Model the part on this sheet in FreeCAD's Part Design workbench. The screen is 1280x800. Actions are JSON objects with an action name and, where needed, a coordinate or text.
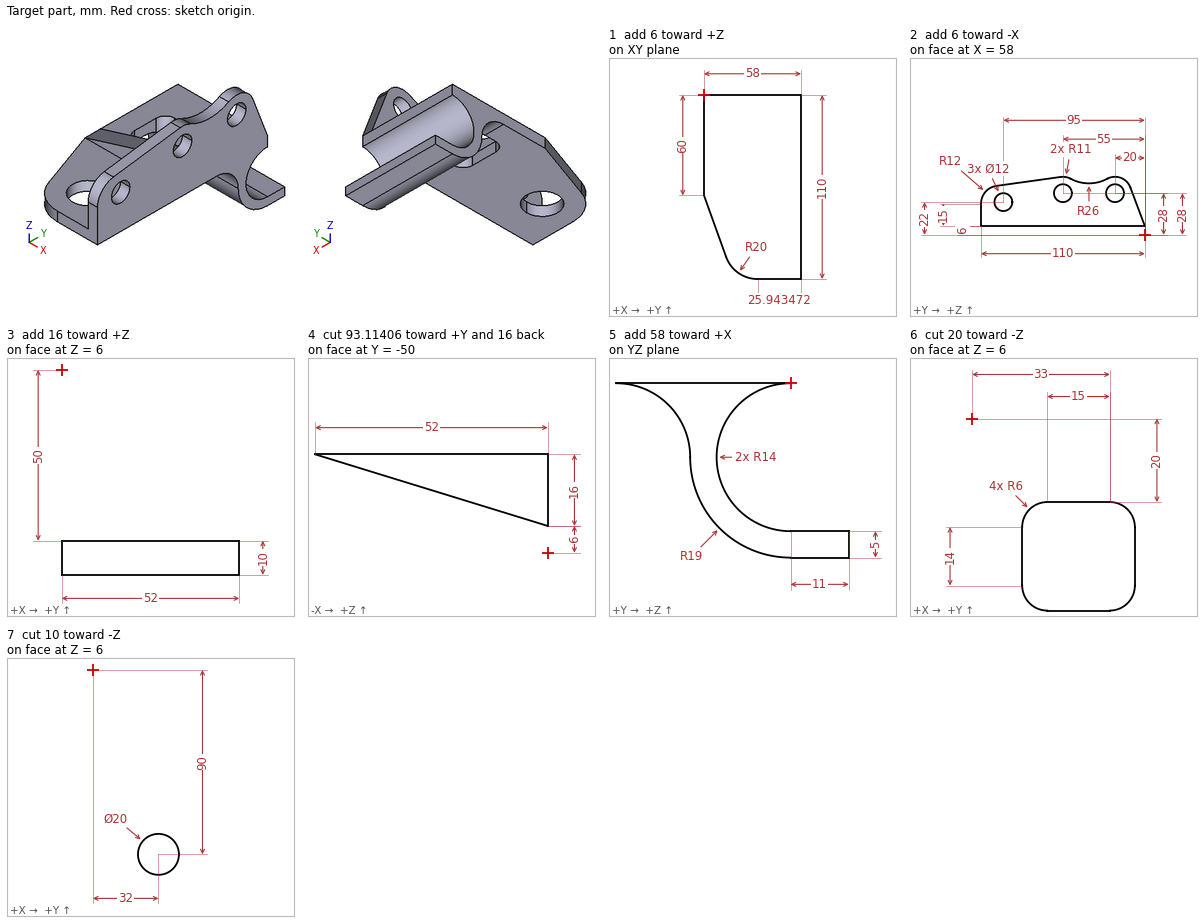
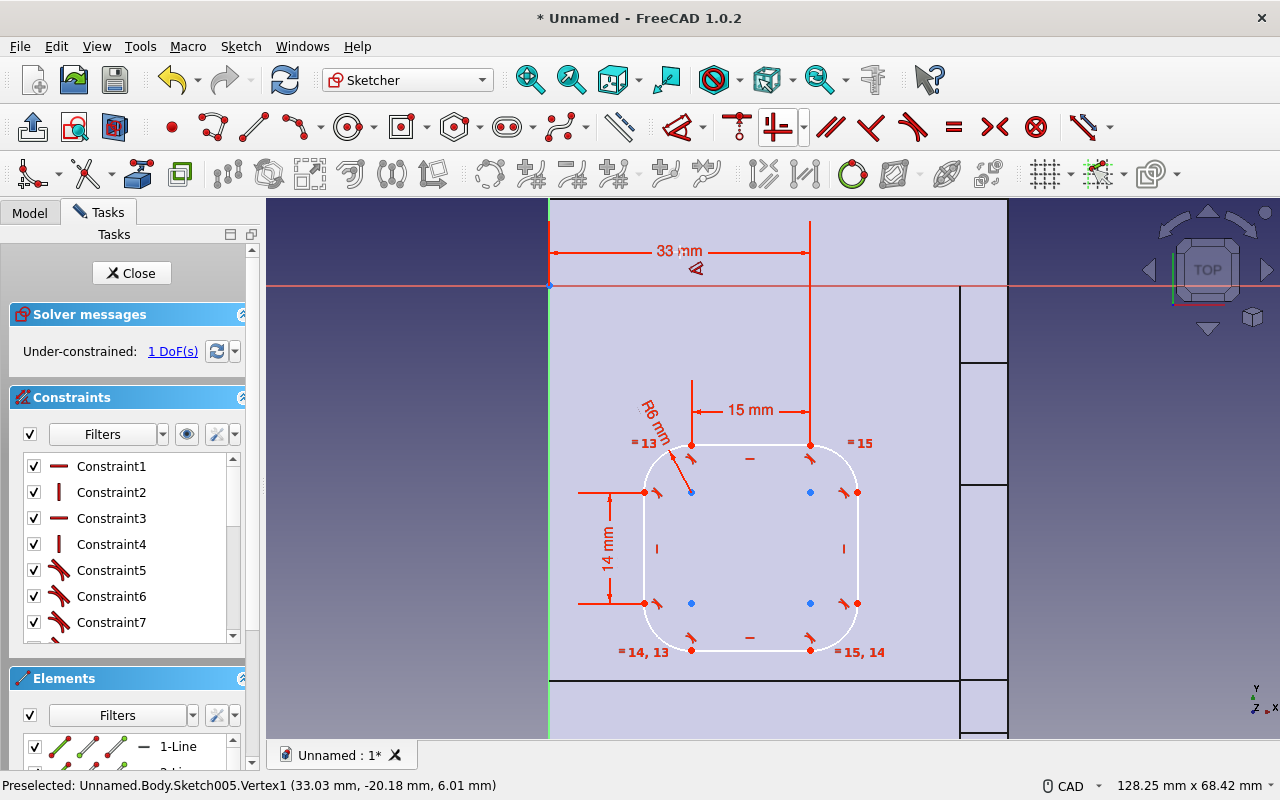
{"action": "left_click", "coordinate": [810, 445]}
{"action": "left_click", "coordinate": [515, 366]}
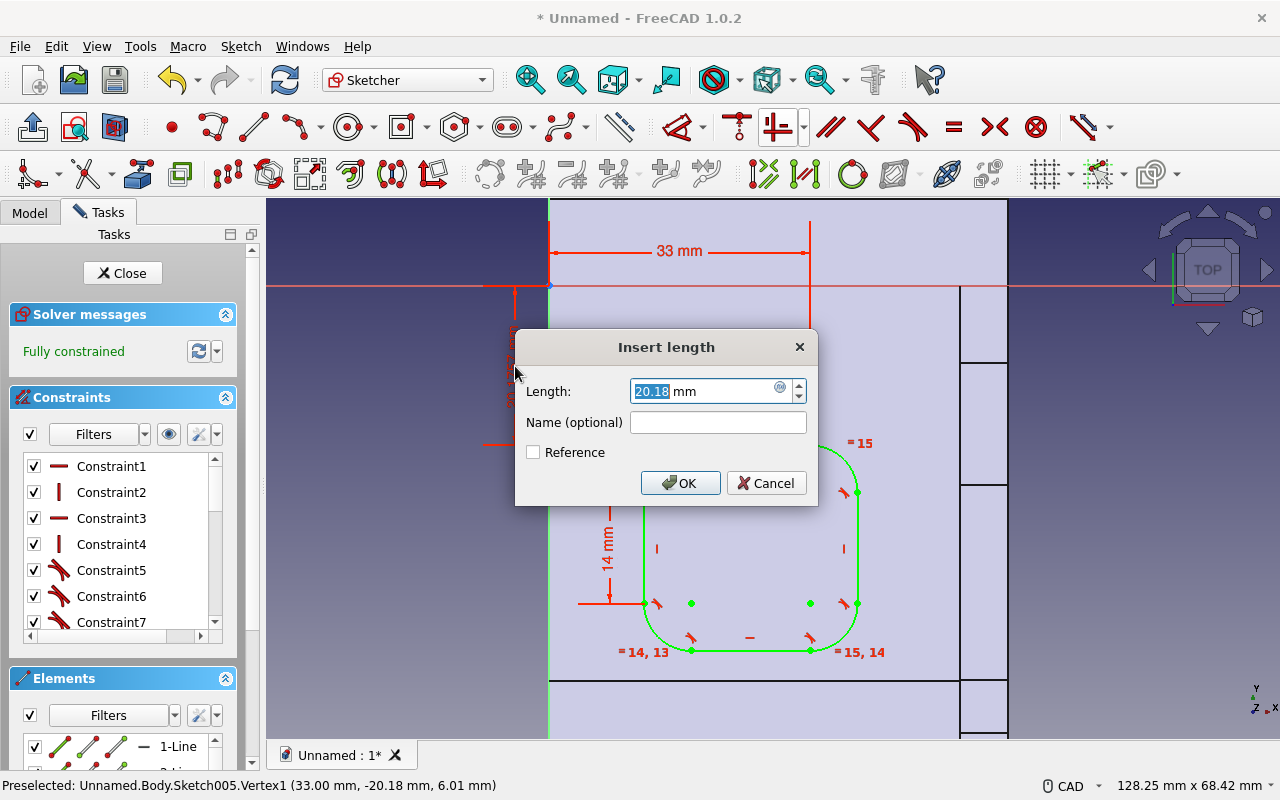
{"action": "type", "text": "20"}
{"action": "key", "text": "Return"}
{"action": "key", "text": "Escape"}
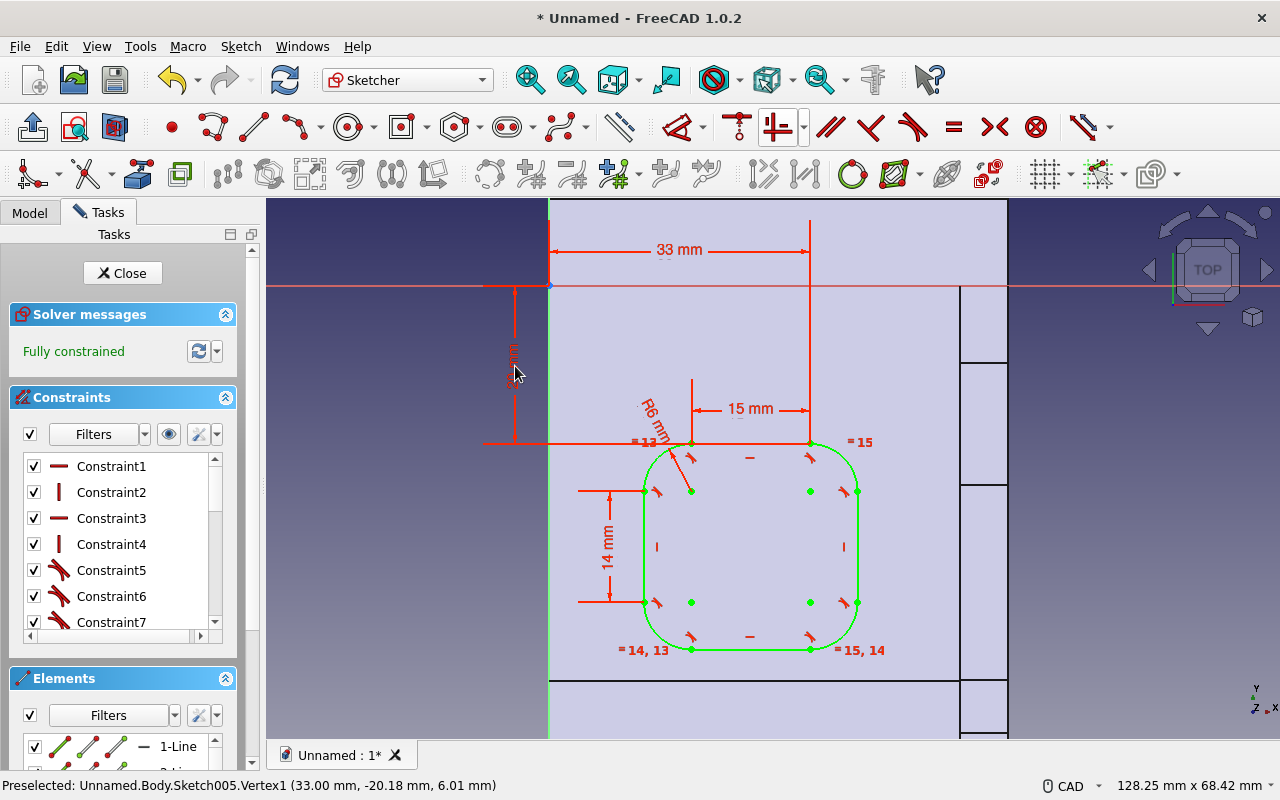
{"action": "left_click", "coordinate": [123, 273]}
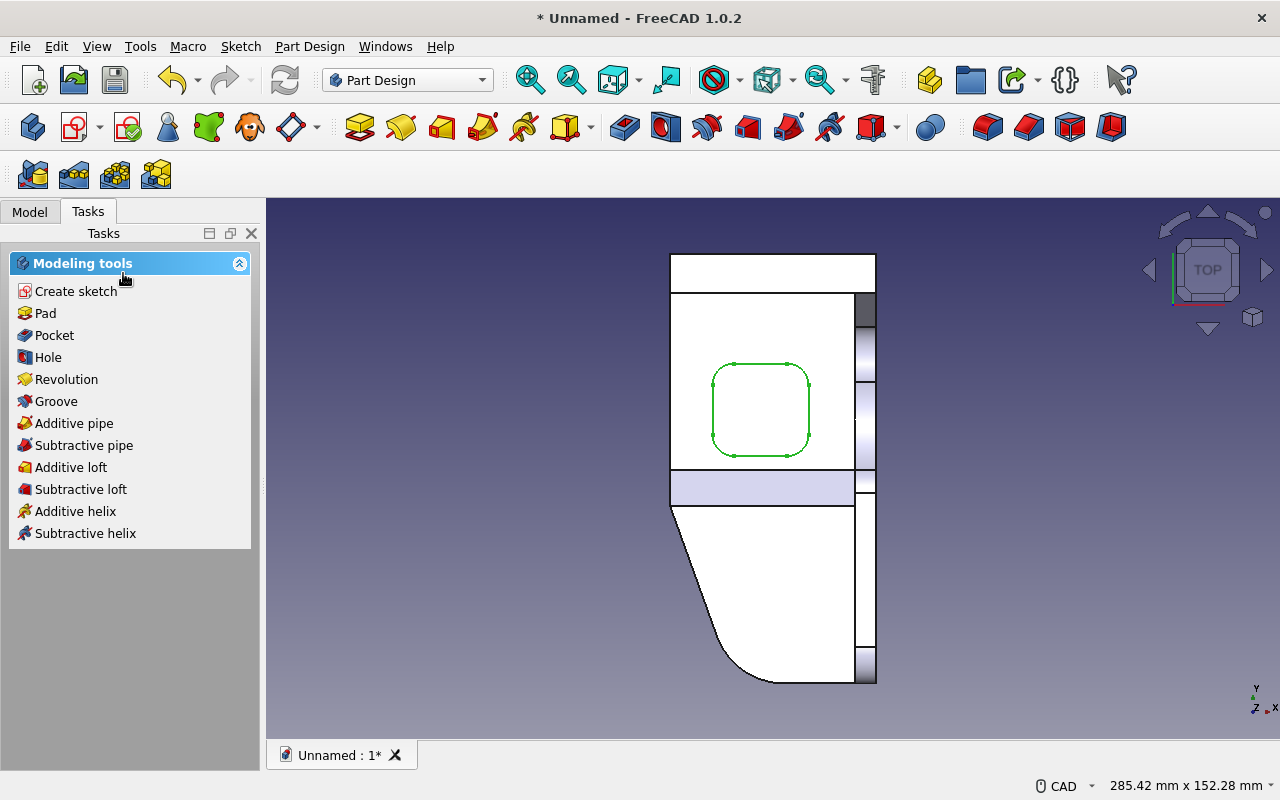
{"action": "left_click", "coordinate": [625, 128]}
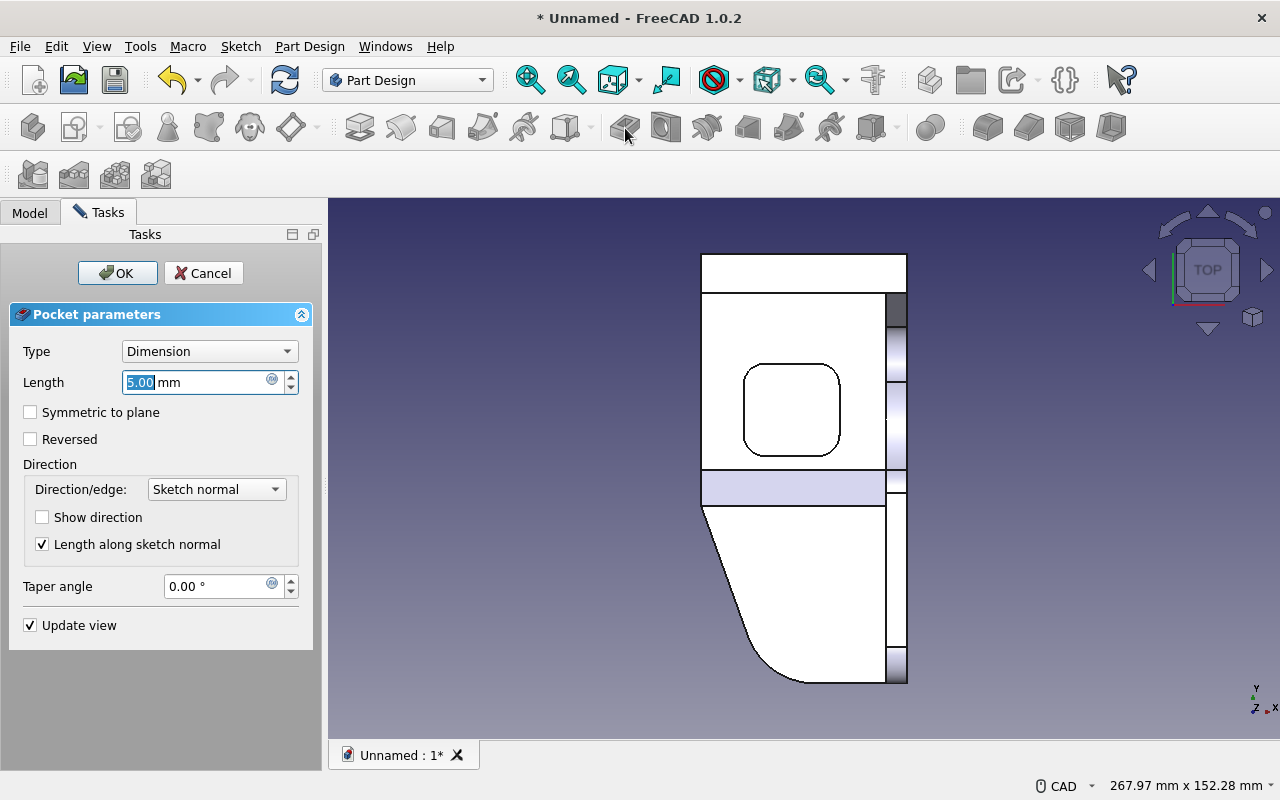
{"action": "type", "text": "20"}
{"action": "key", "text": "Tab"}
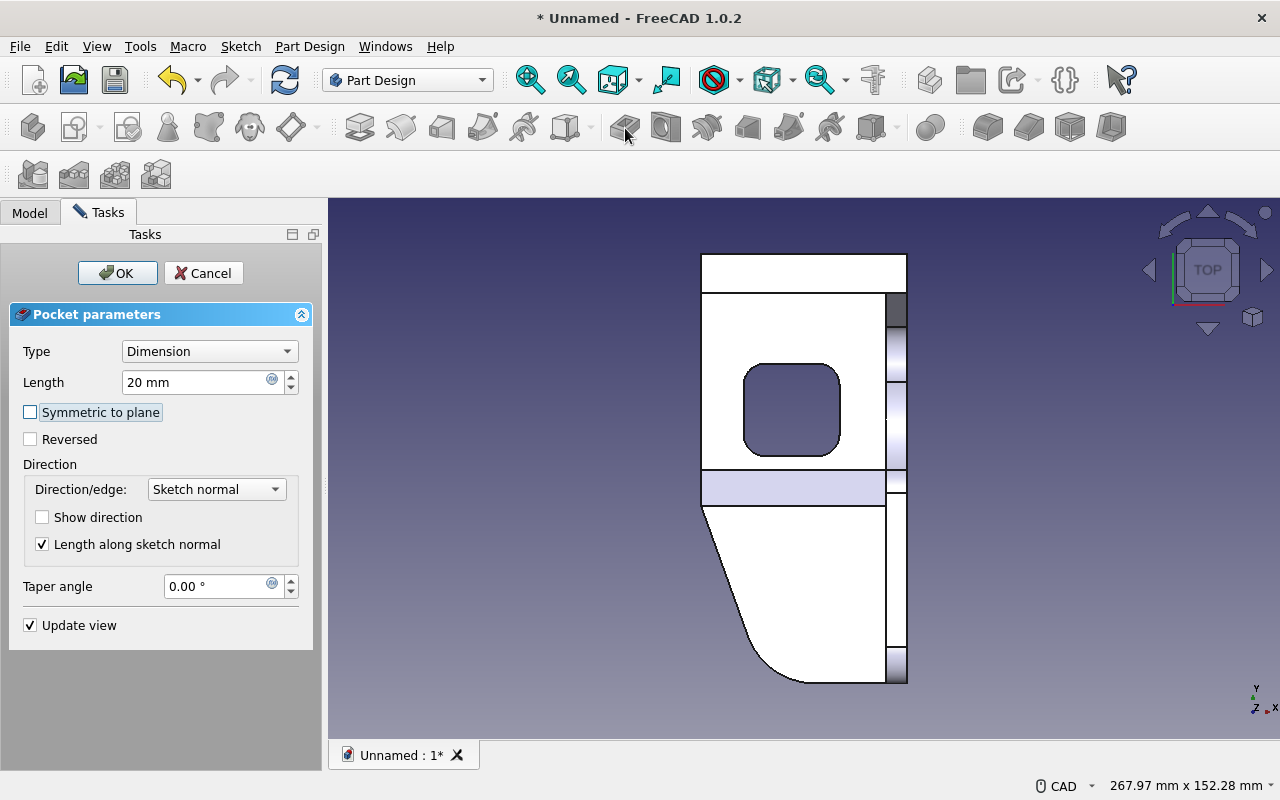
{"action": "left_click", "coordinate": [118, 273]}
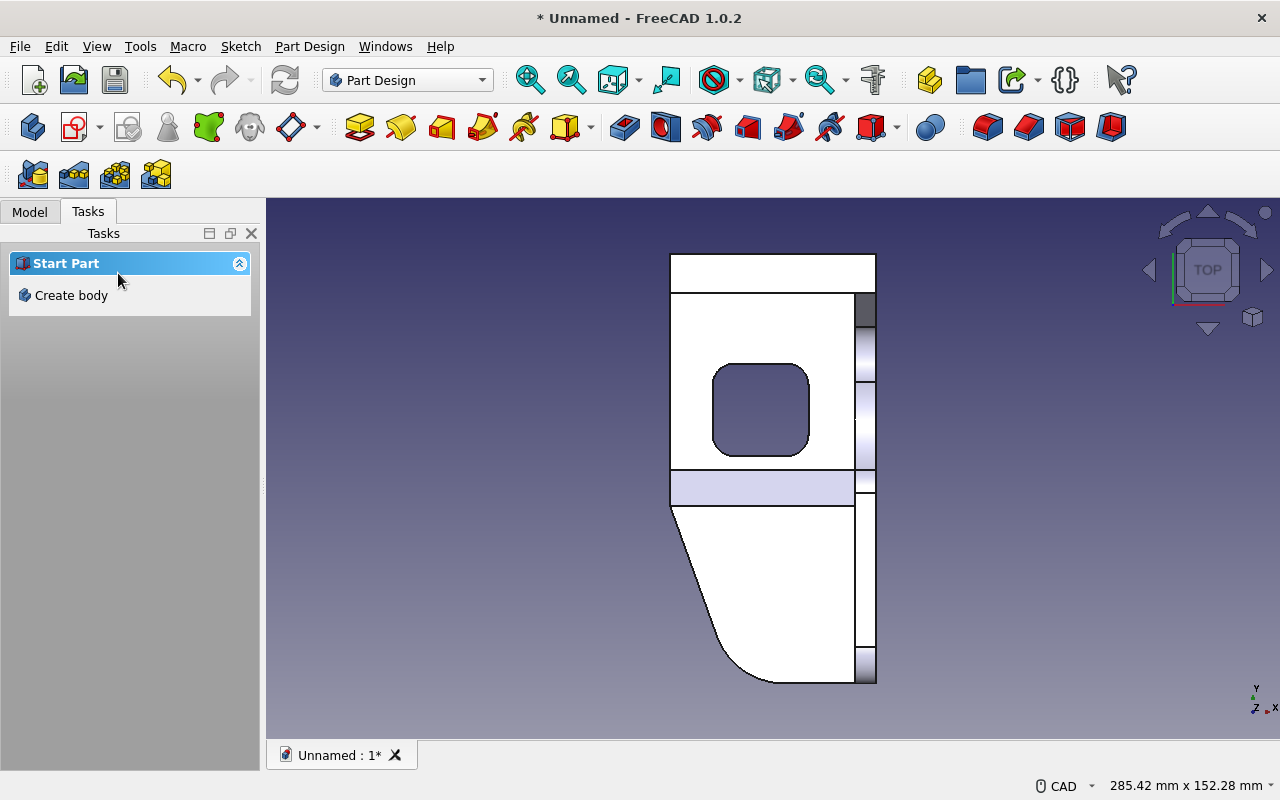
{"action": "left_click", "coordinate": [789, 594]}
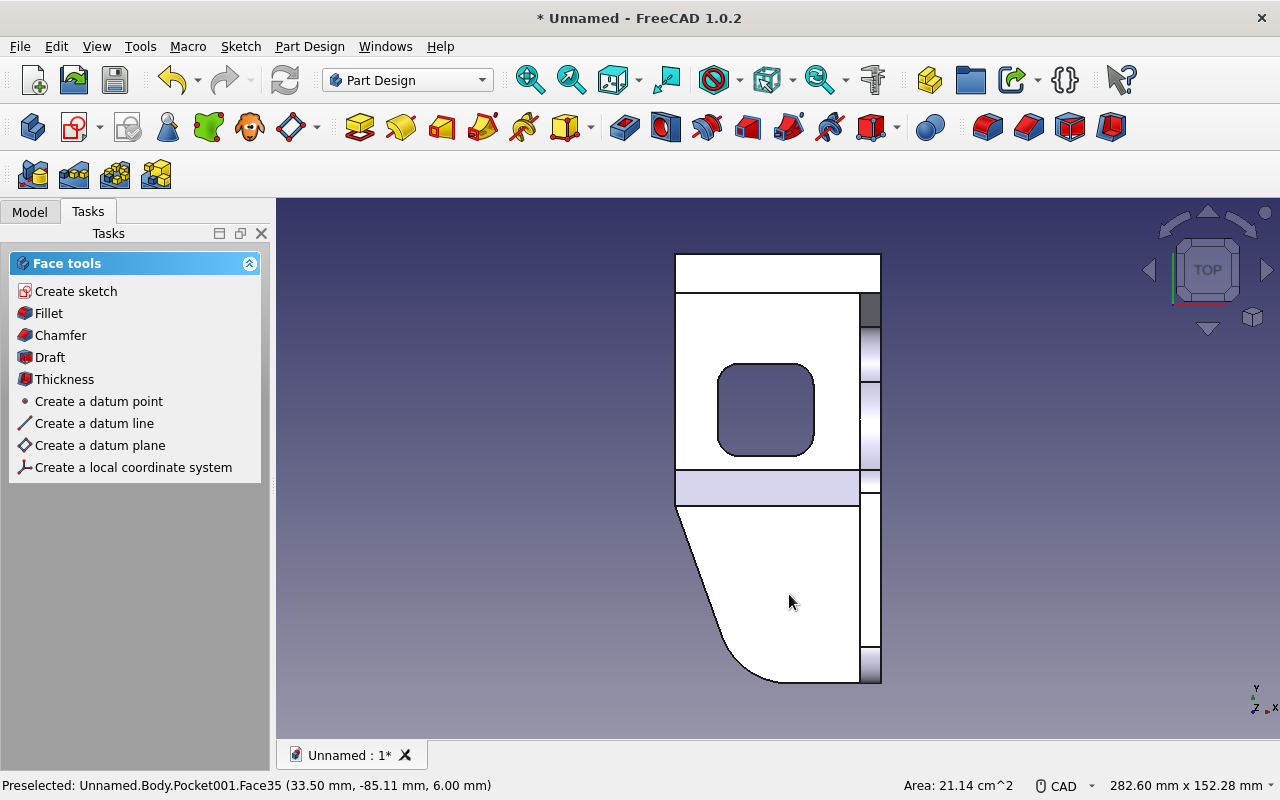
{"action": "left_click", "coordinate": [74, 128]}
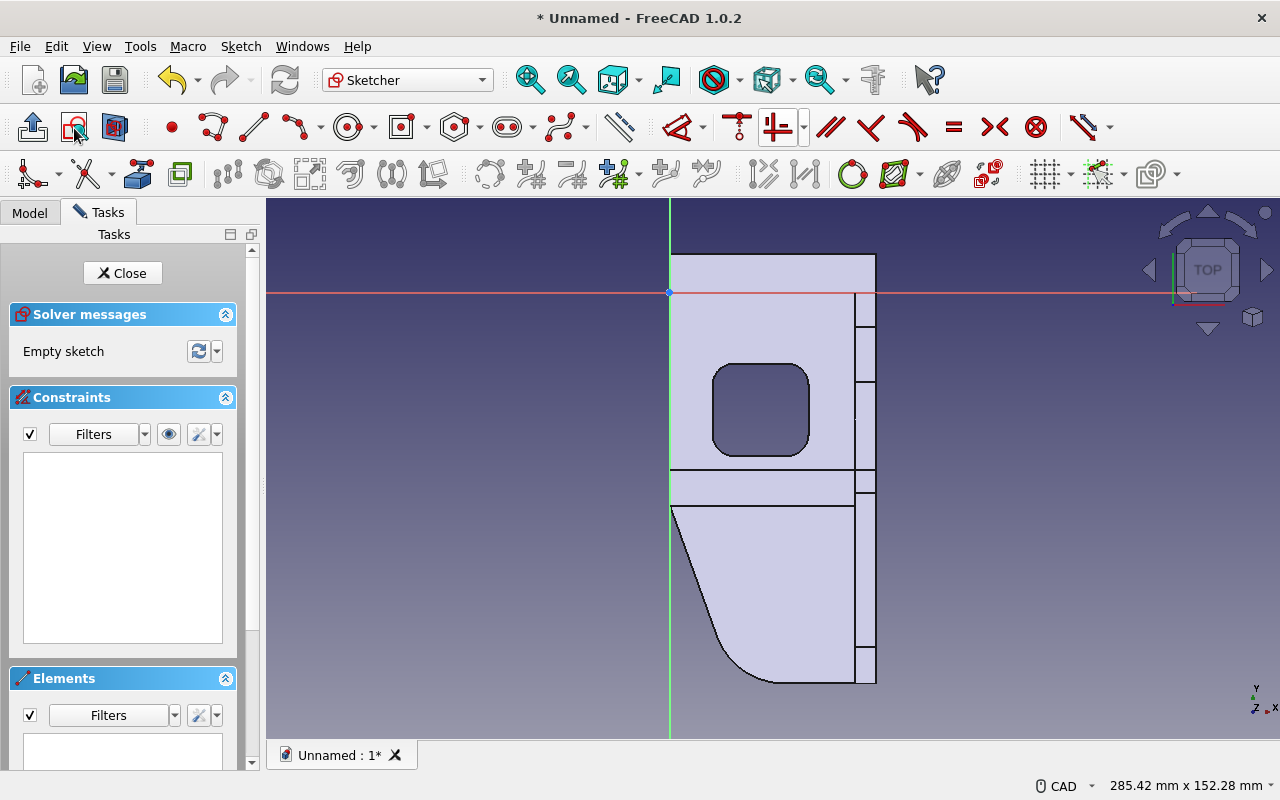
{"action": "scroll", "coordinate": [804, 649], "scroll_direction": "up", "scroll_amount": 8}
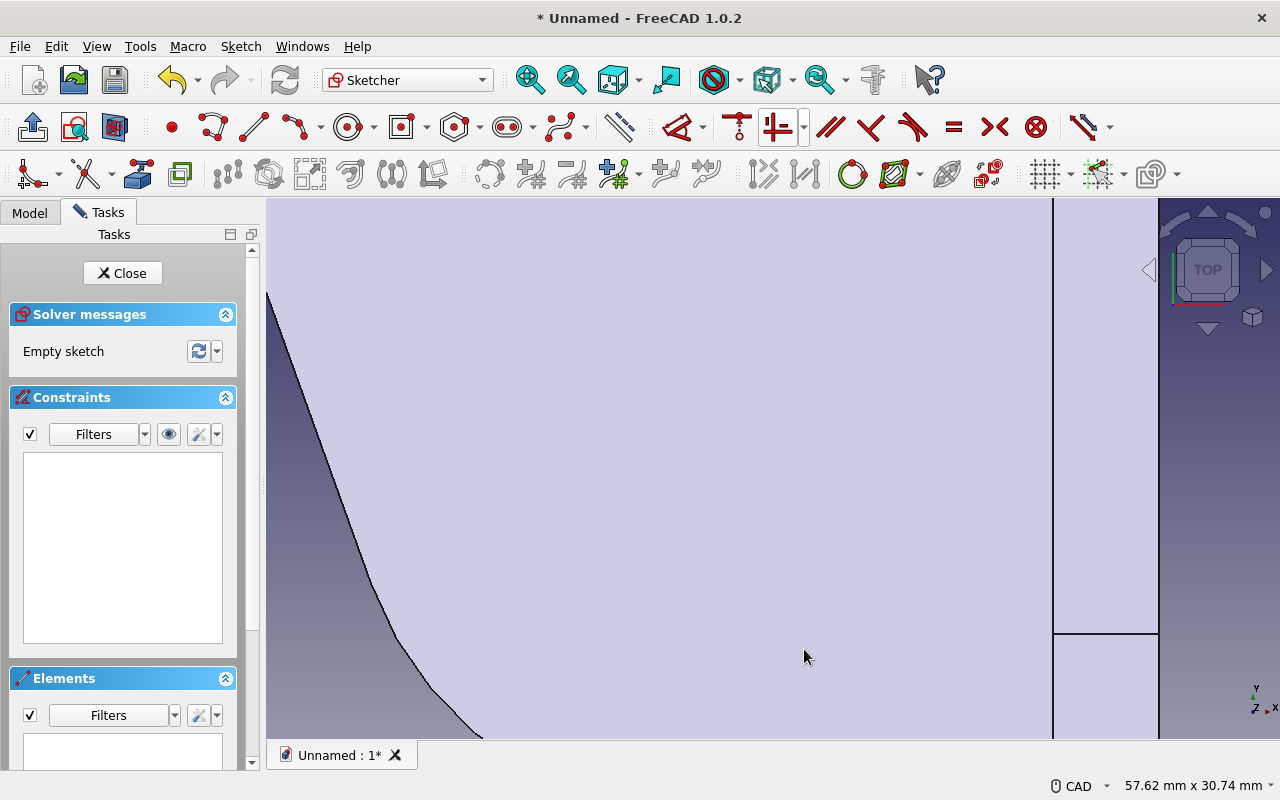
{"action": "left_click", "coordinate": [348, 128]}